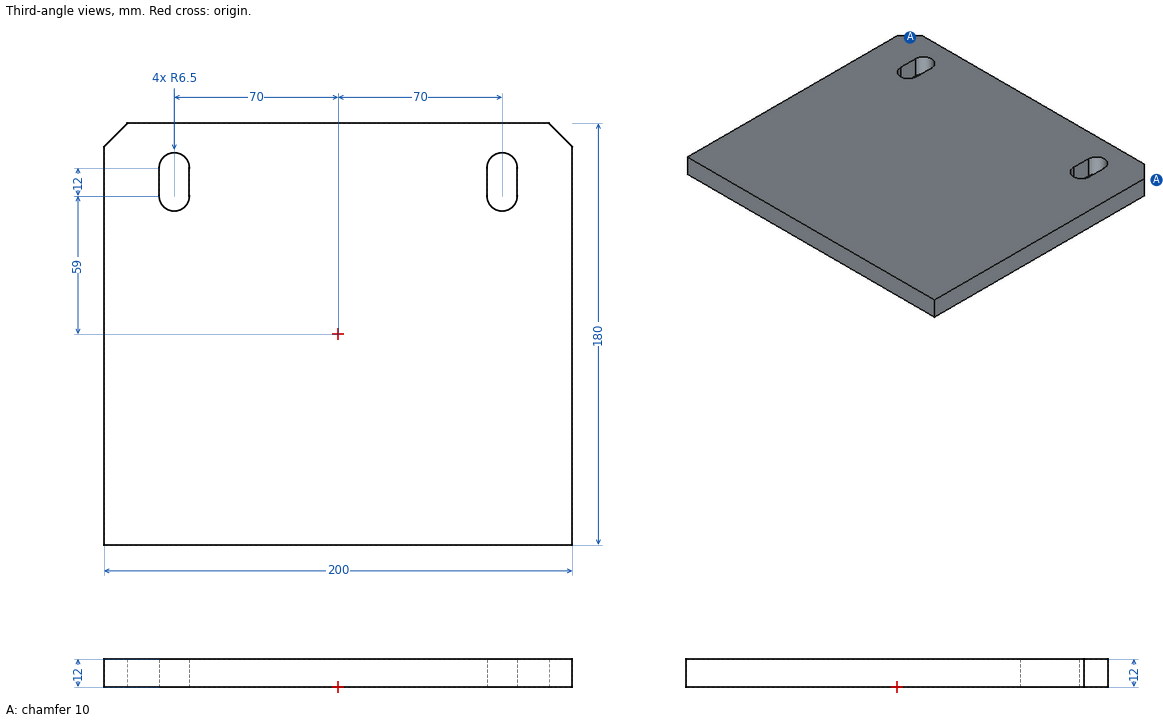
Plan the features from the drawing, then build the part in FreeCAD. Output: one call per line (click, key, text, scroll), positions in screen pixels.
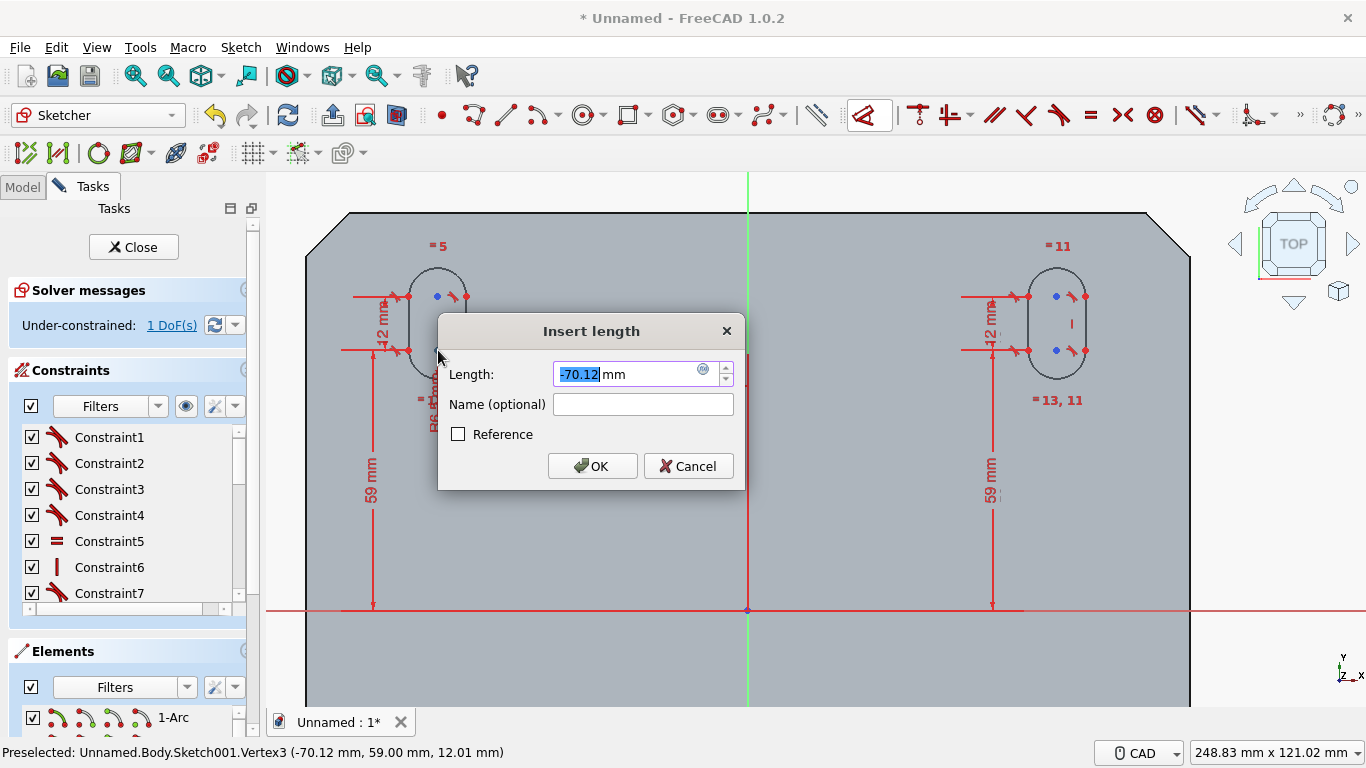
text(-70)
key(Return)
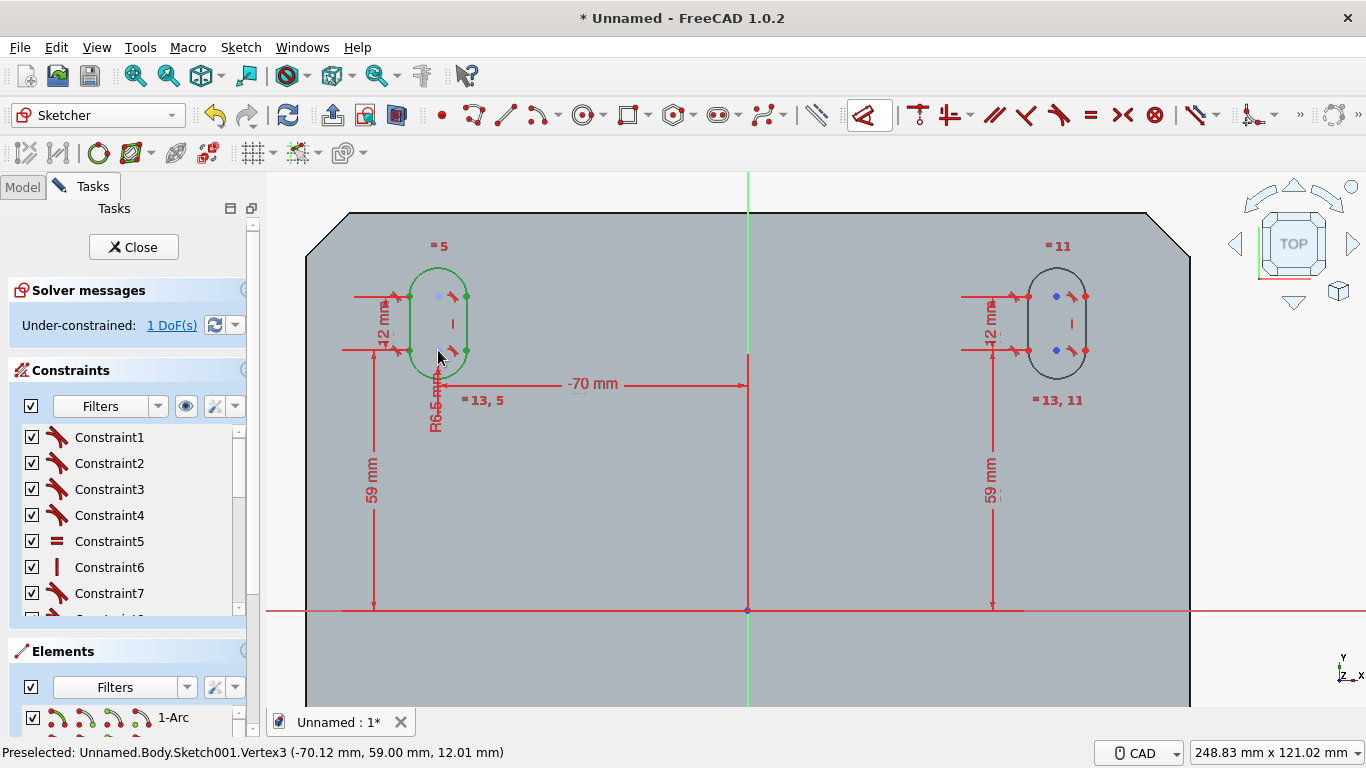
click(1057, 350)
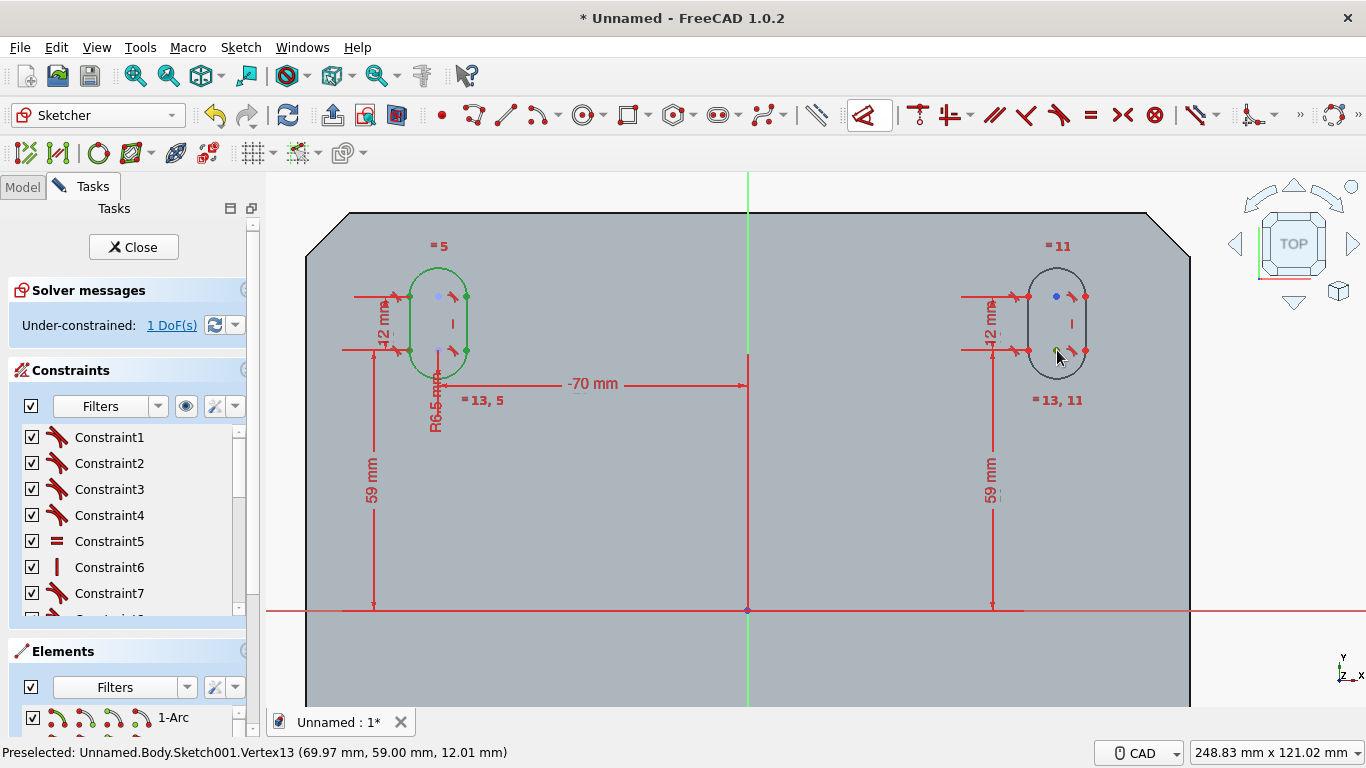
key(l)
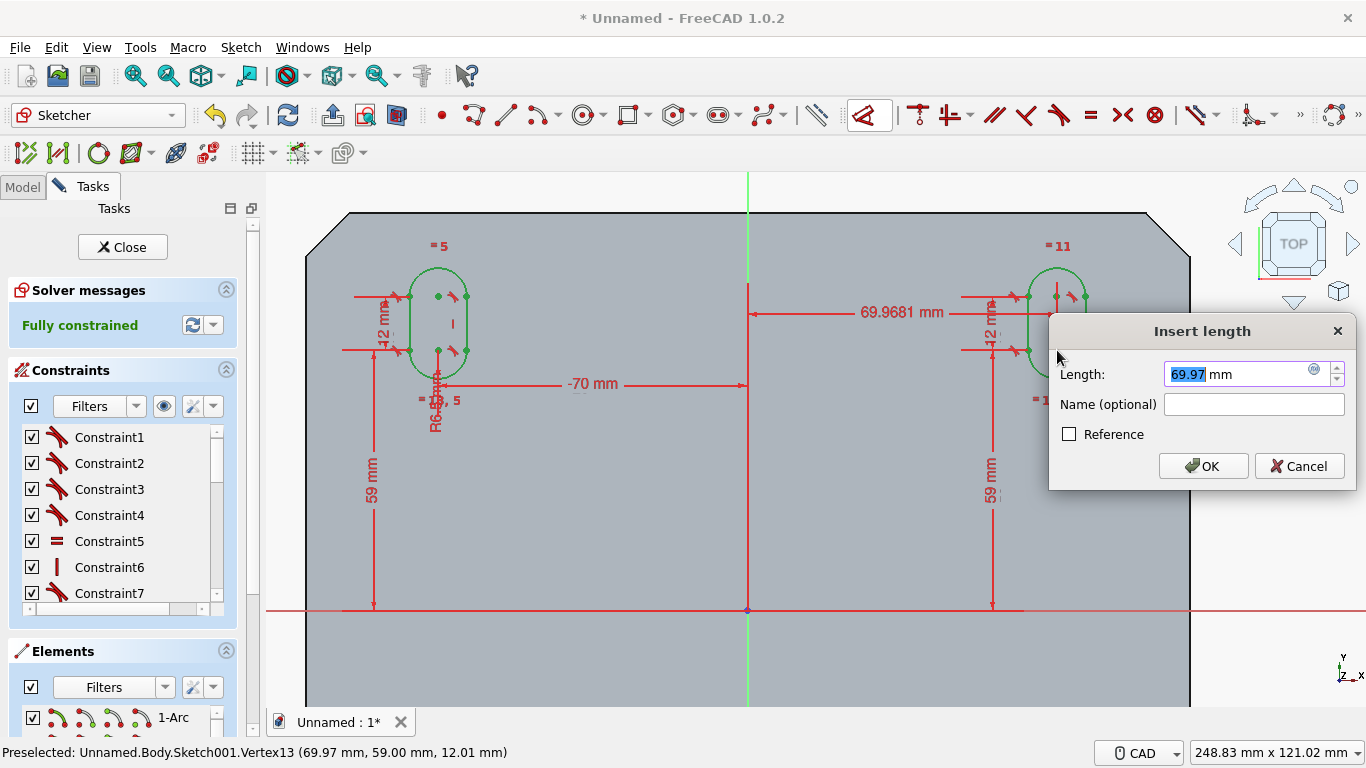
text(70)
key(Return)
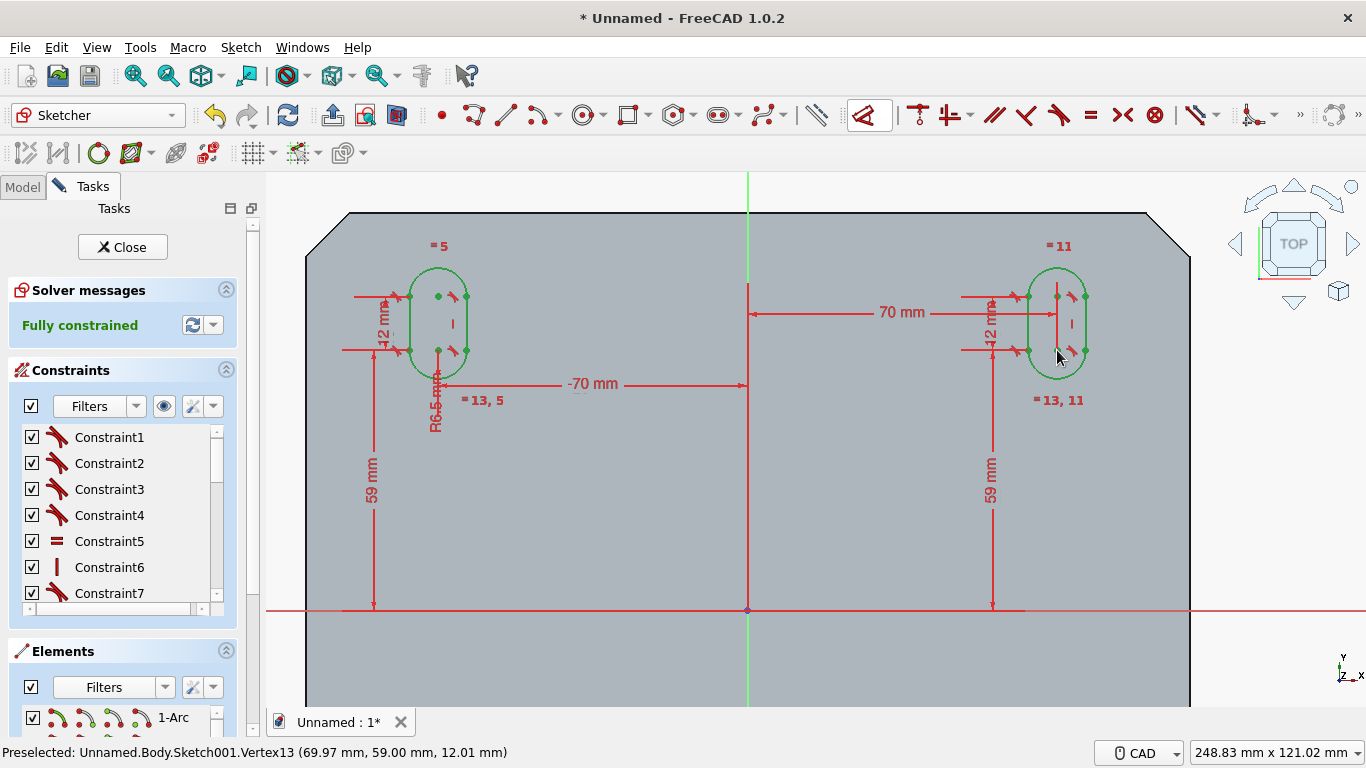
click(123, 247)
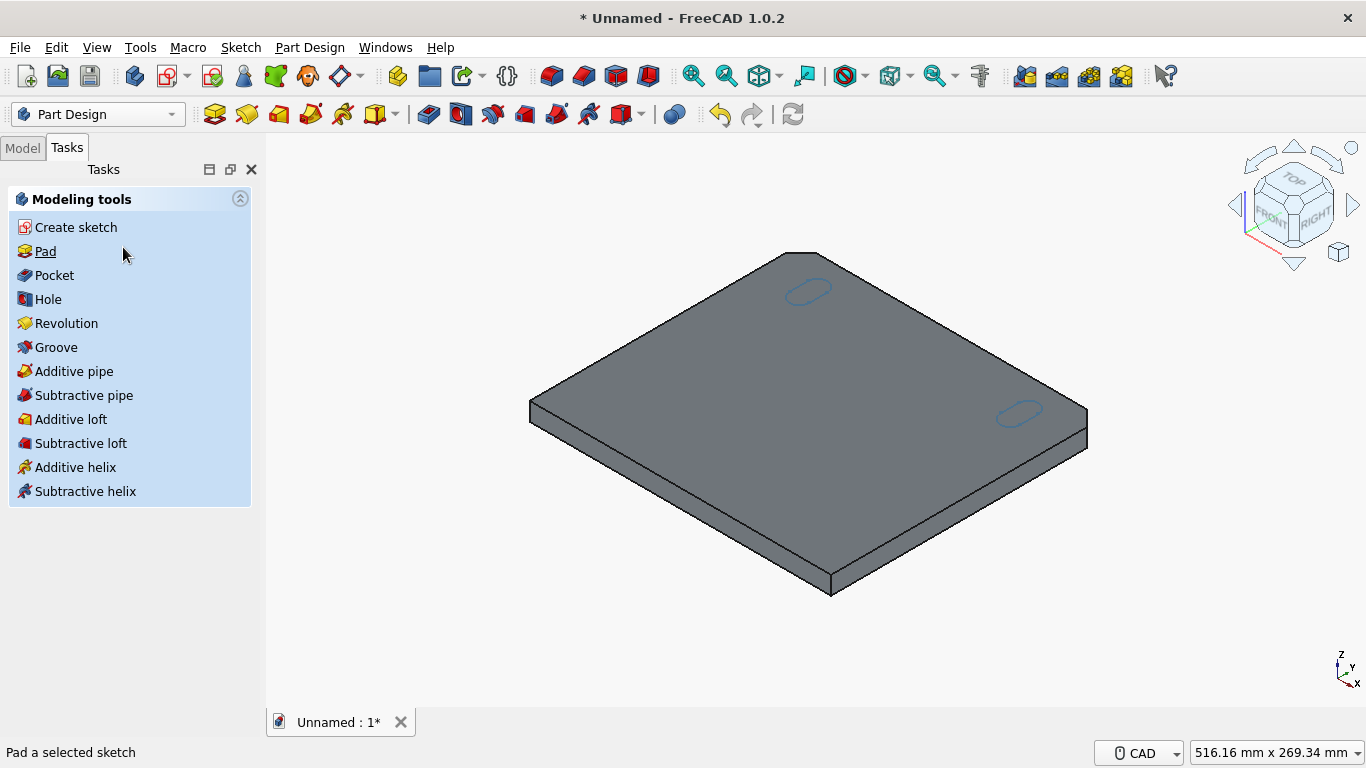
click(430, 114)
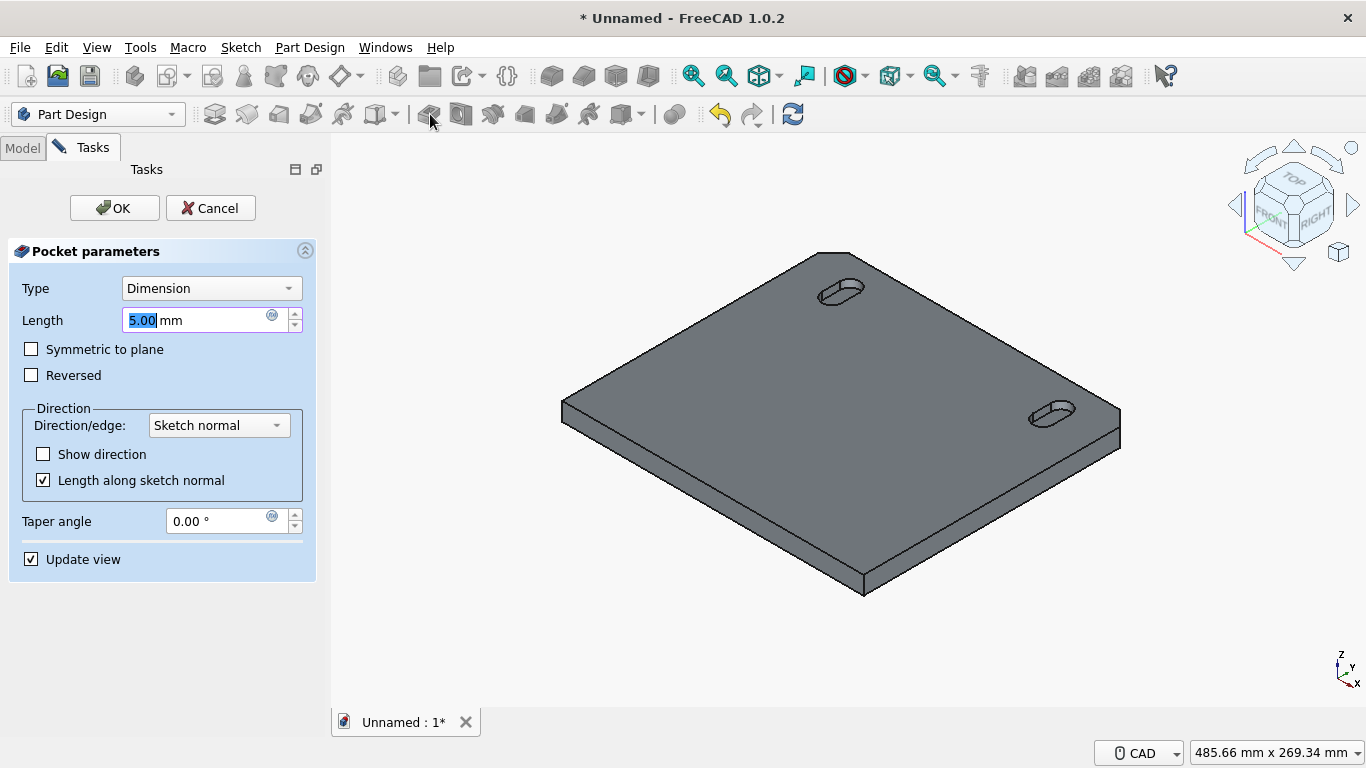
text(12)
key(Tab)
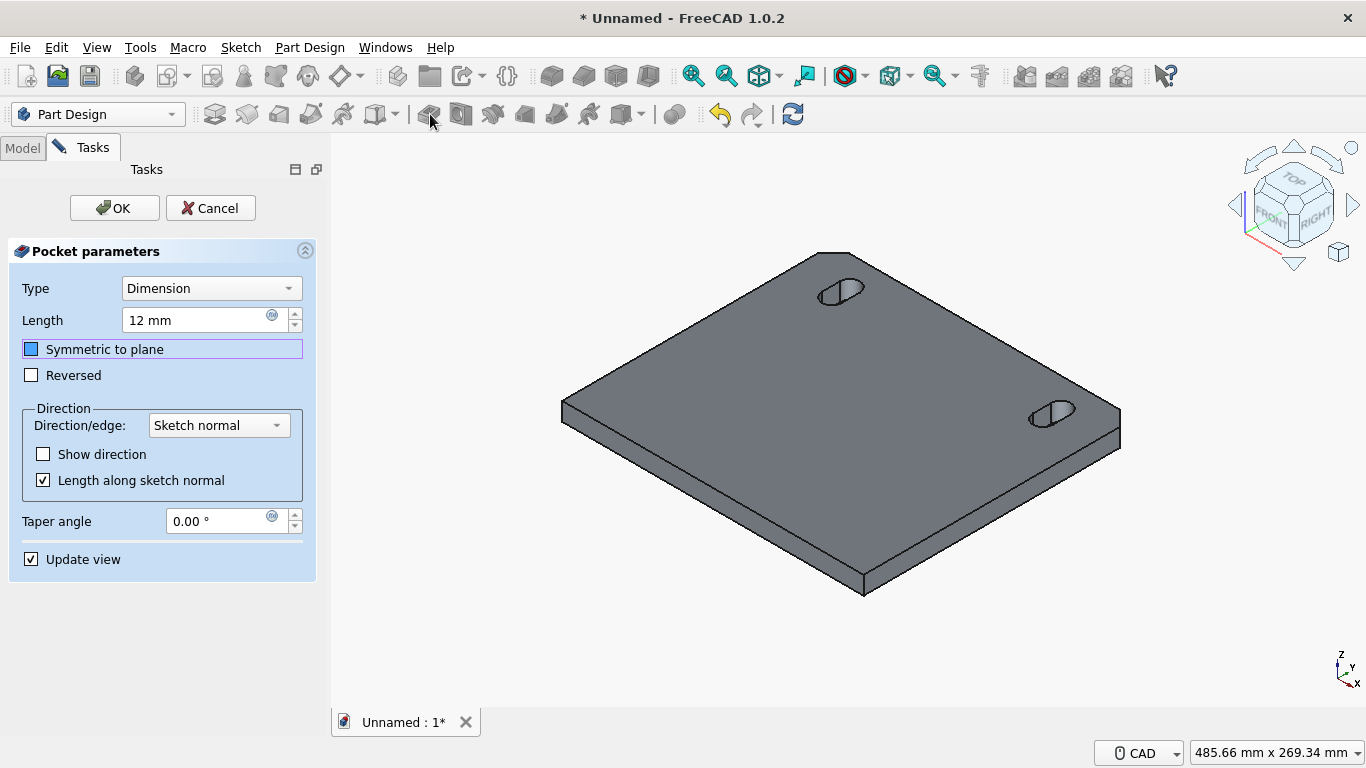
click(115, 208)